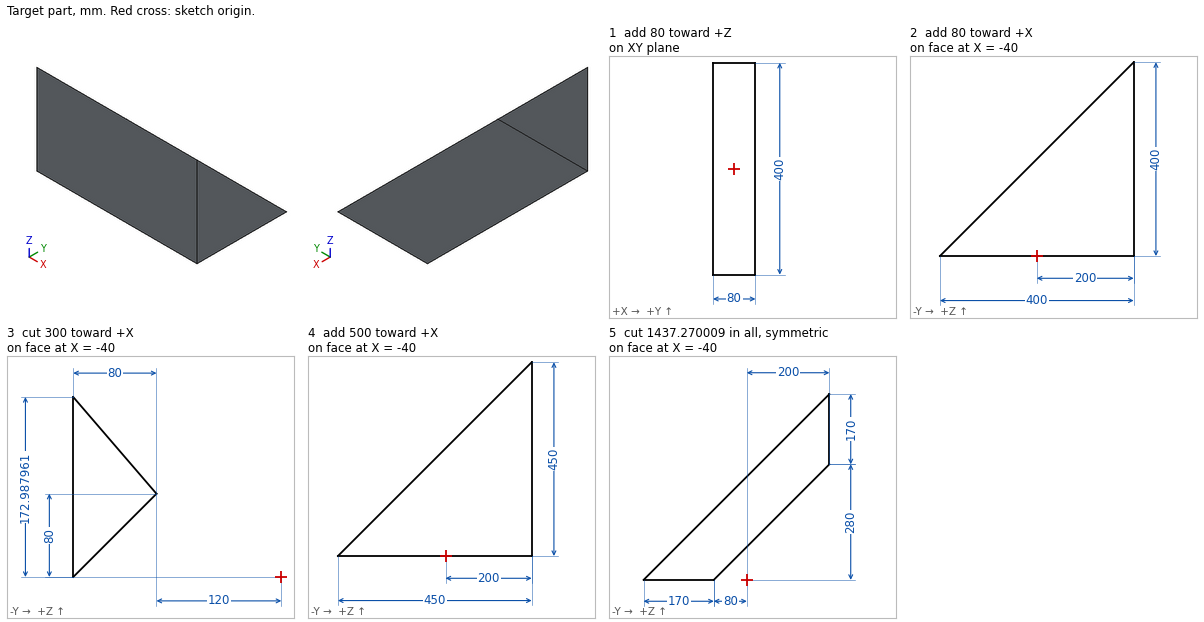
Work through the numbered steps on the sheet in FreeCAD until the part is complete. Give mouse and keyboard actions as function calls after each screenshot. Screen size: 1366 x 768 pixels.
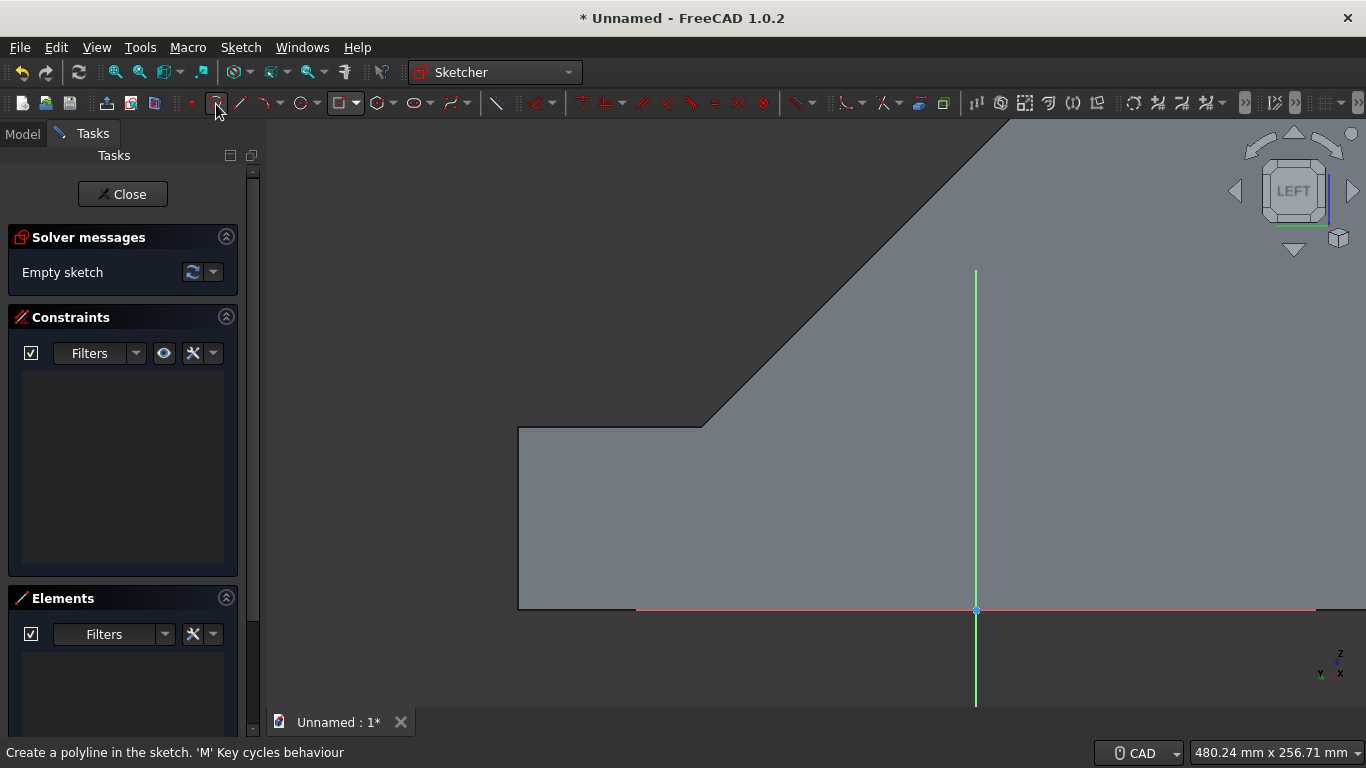
click(701, 427)
click(518, 214)
click(518, 610)
click(701, 428)
key(Escape)
key(Escape)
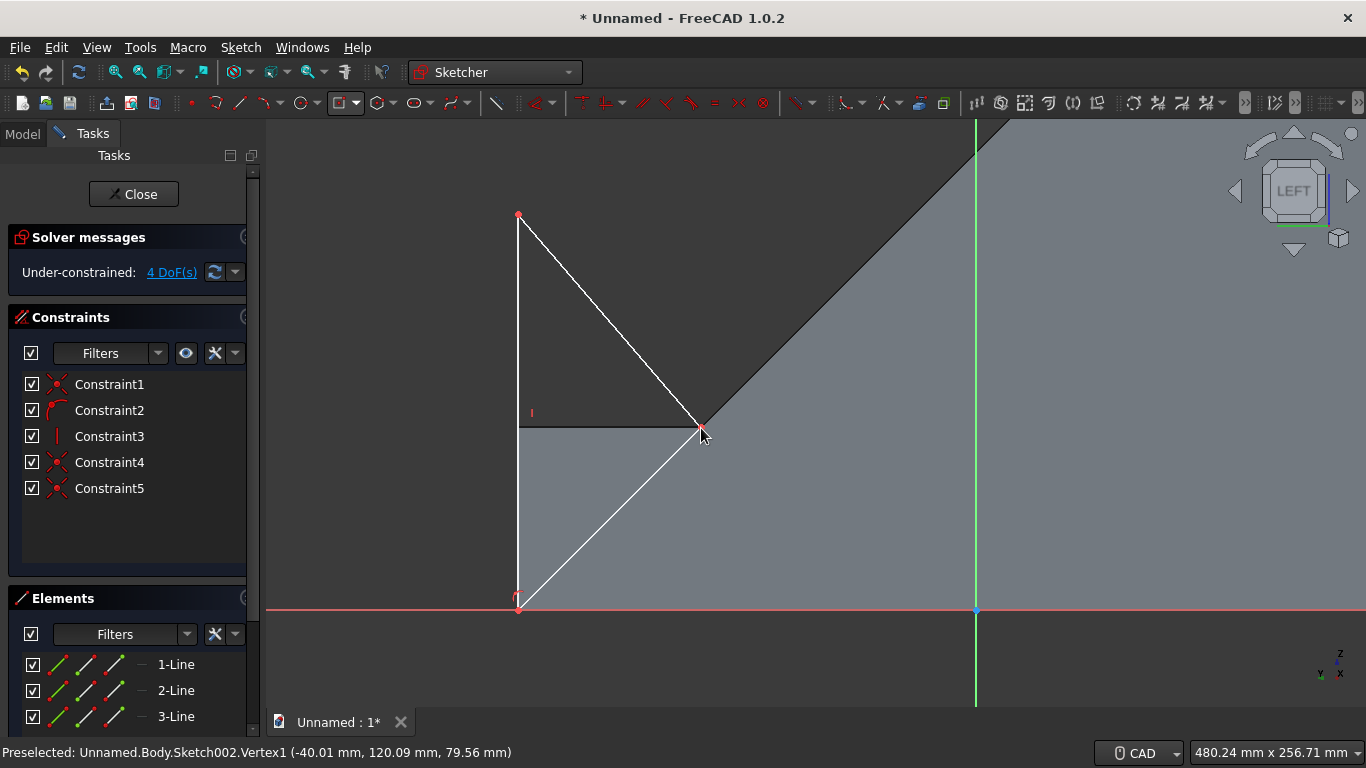
click(536, 104)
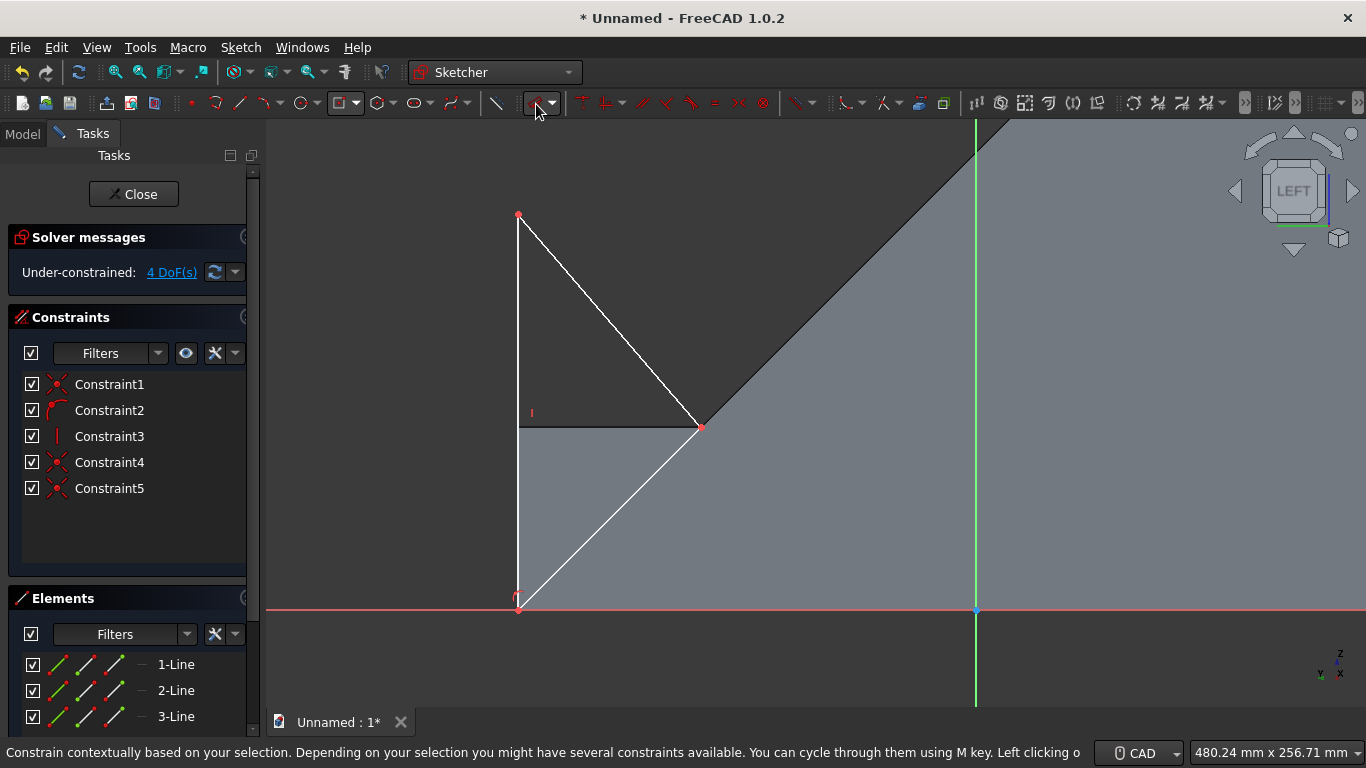
click(701, 428)
click(1010, 519)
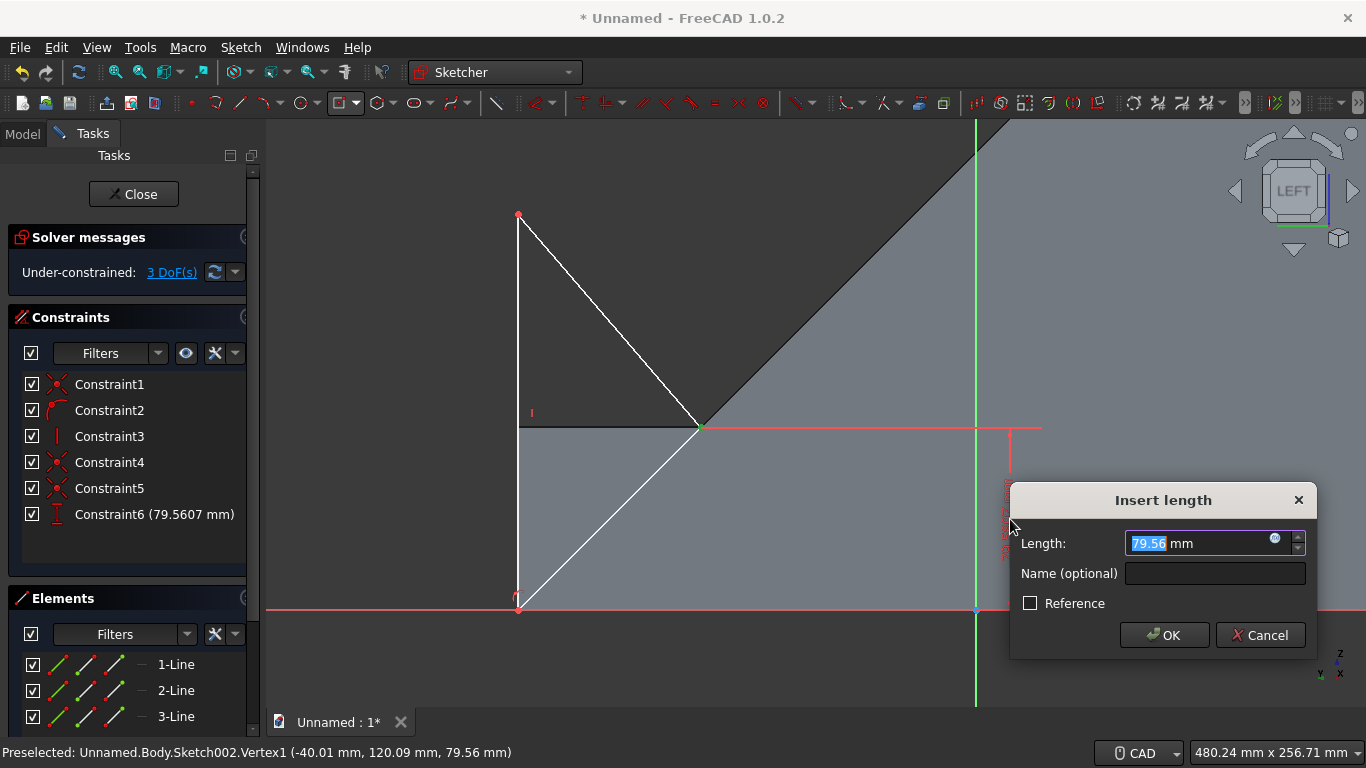
text(80)
key(Return)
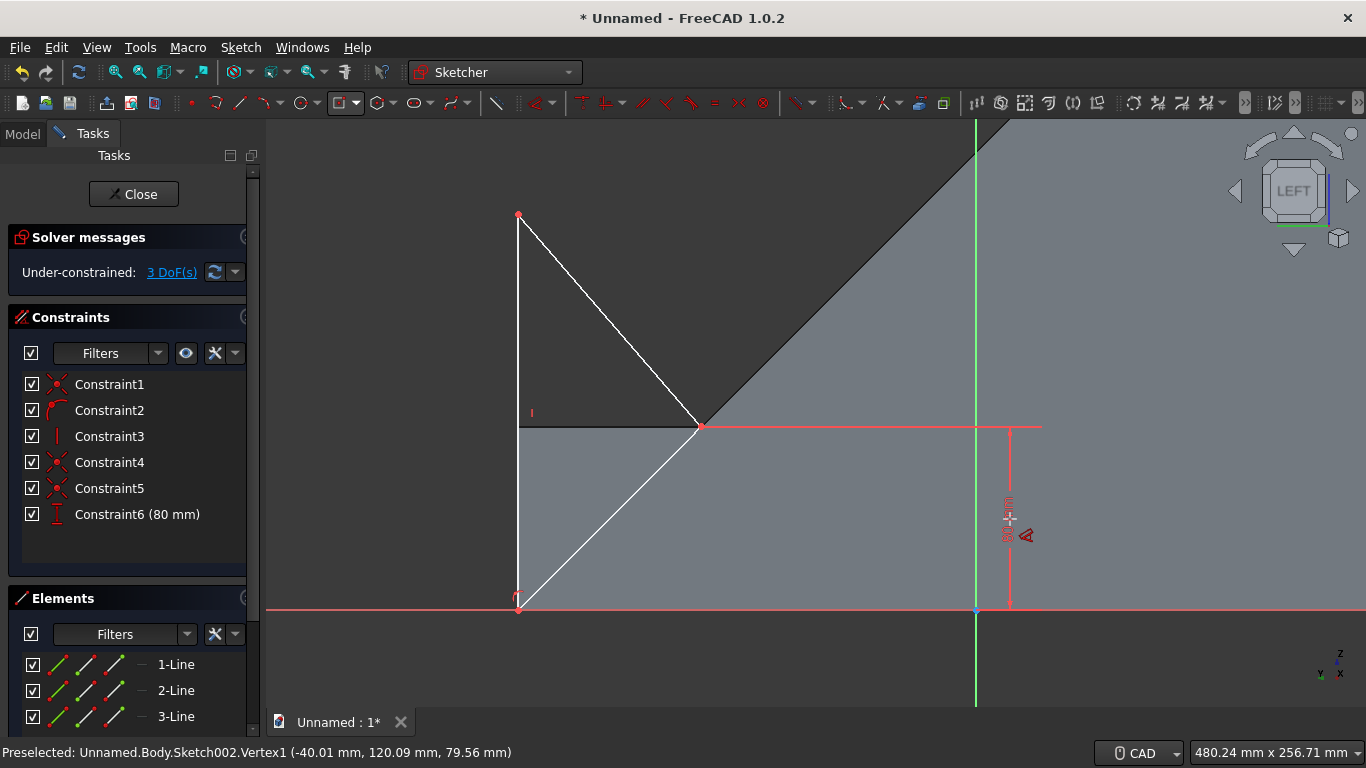
click(646, 363)
click(610, 181)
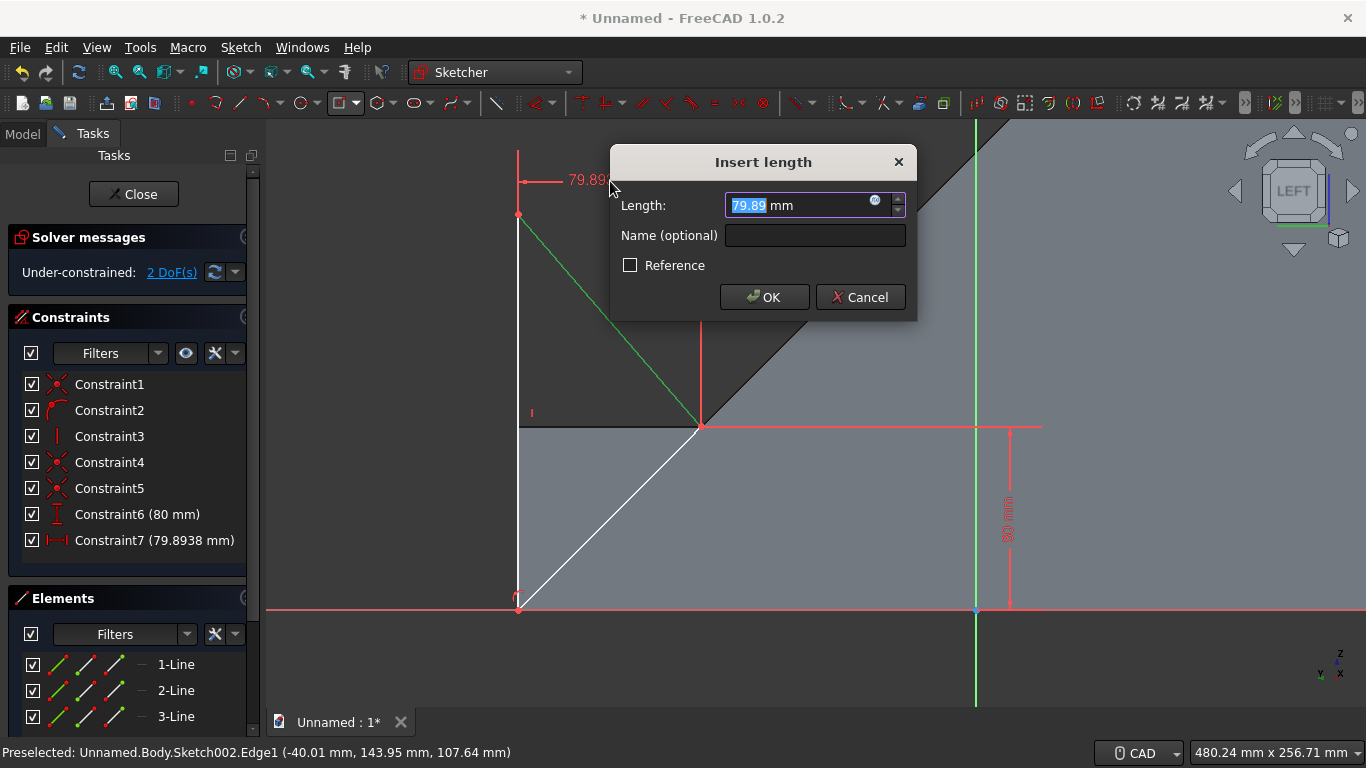
text(80)
key(Return)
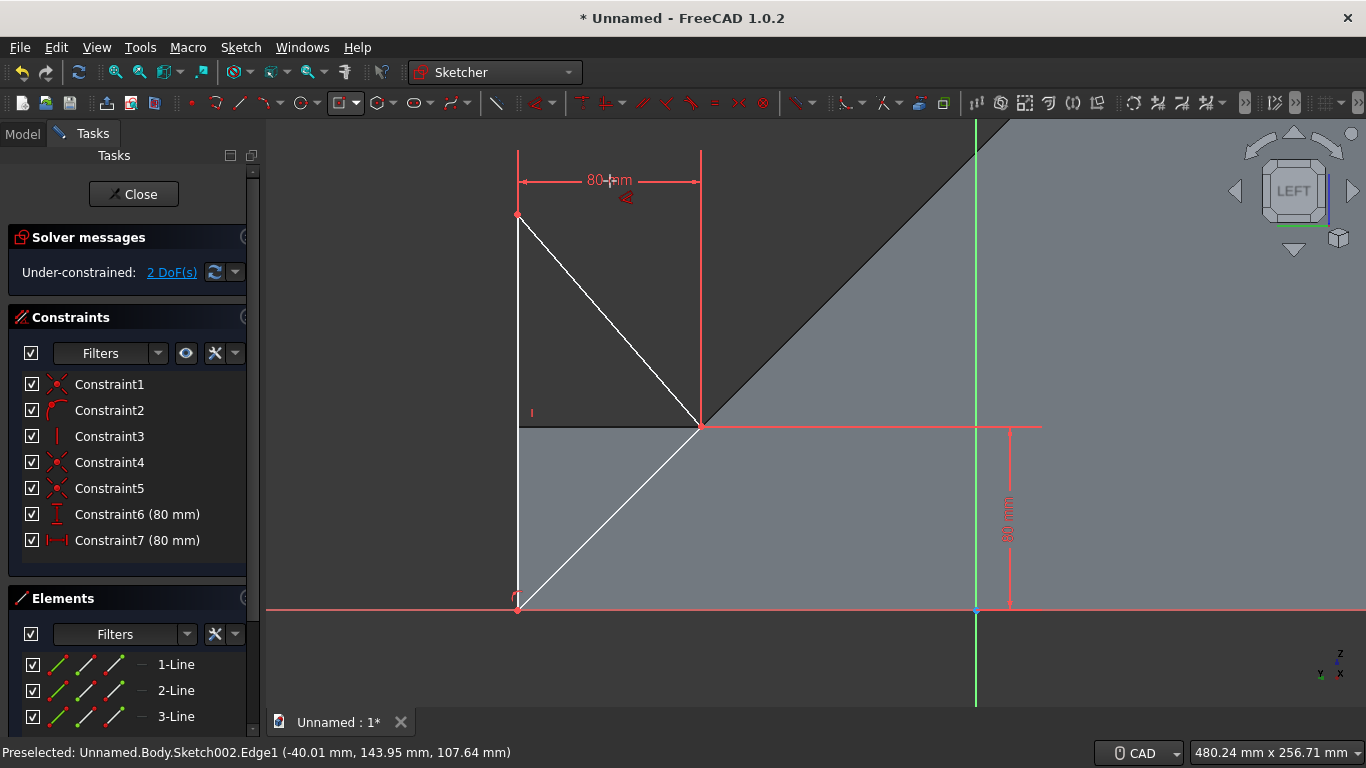
click(701, 427)
click(839, 644)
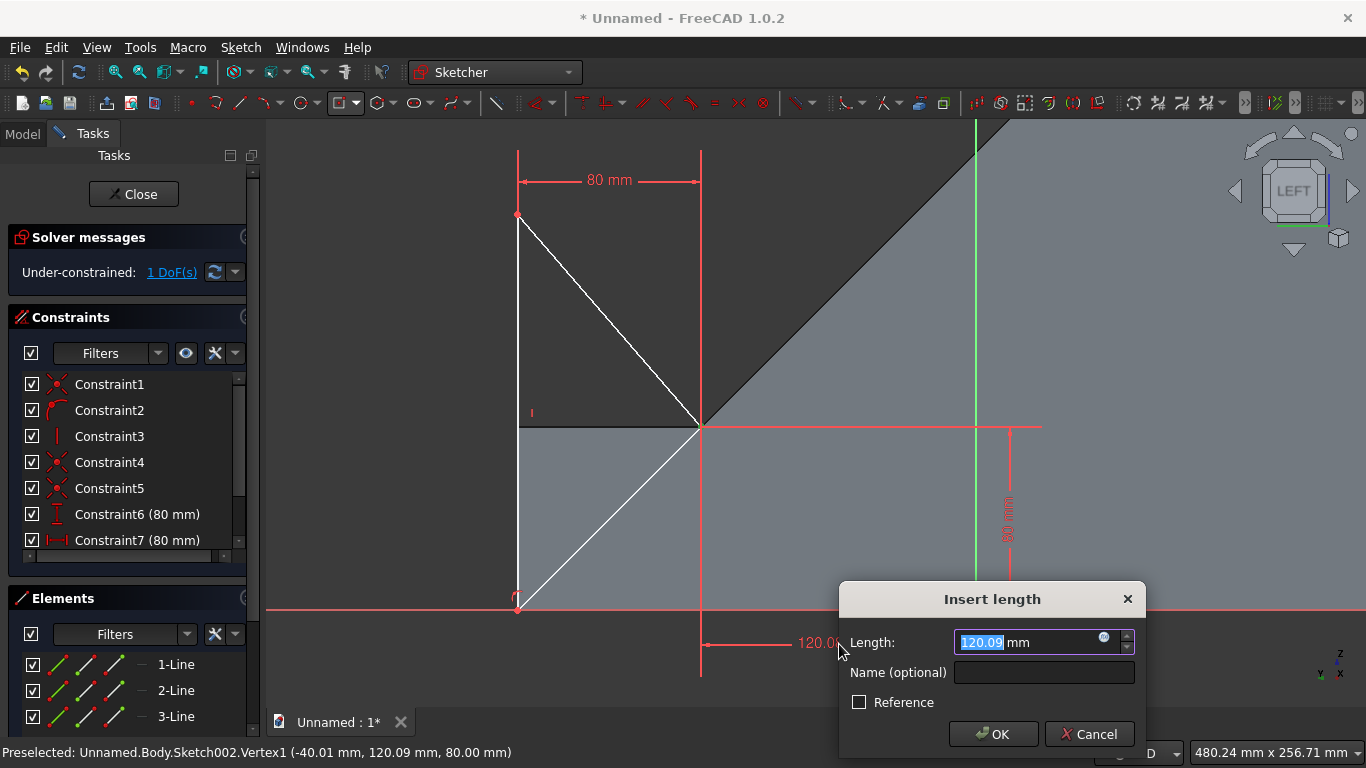
text(120)
key(Return)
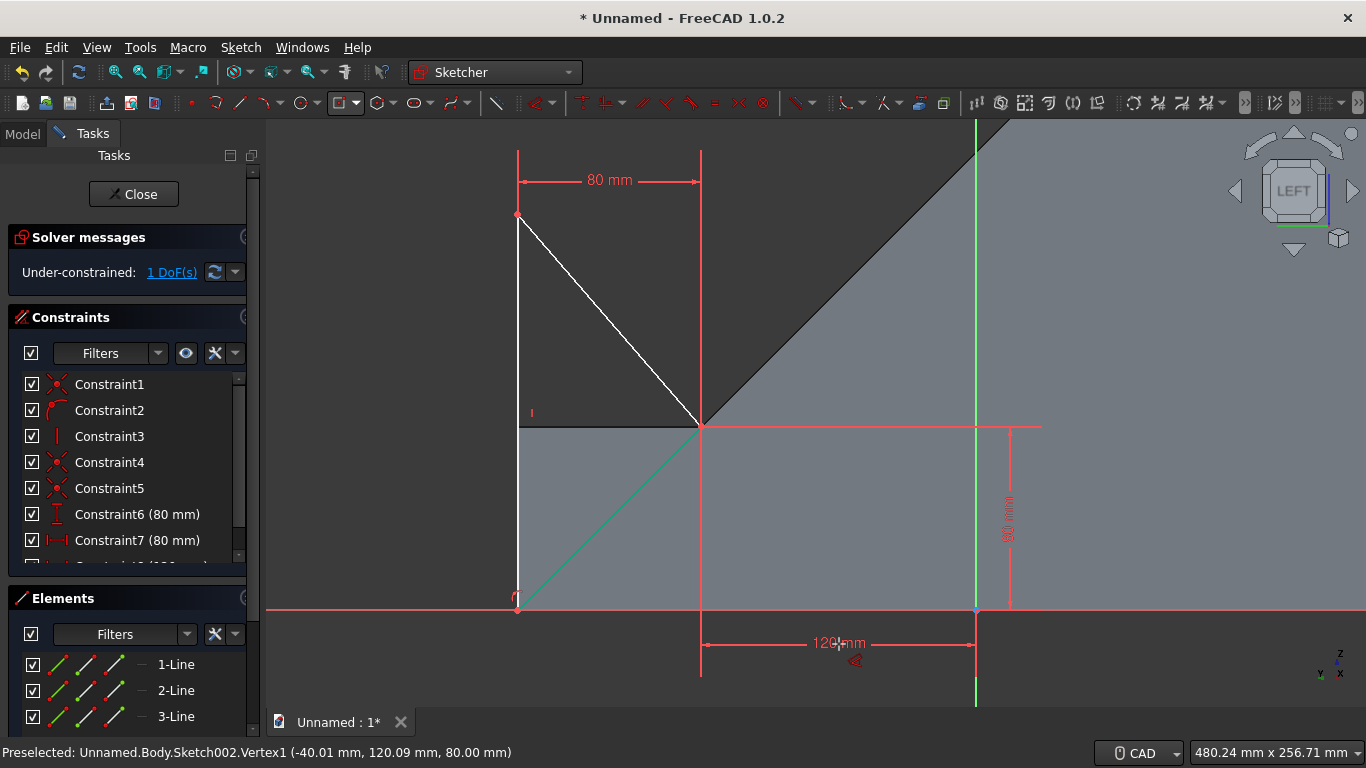
click(518, 334)
click(484, 413)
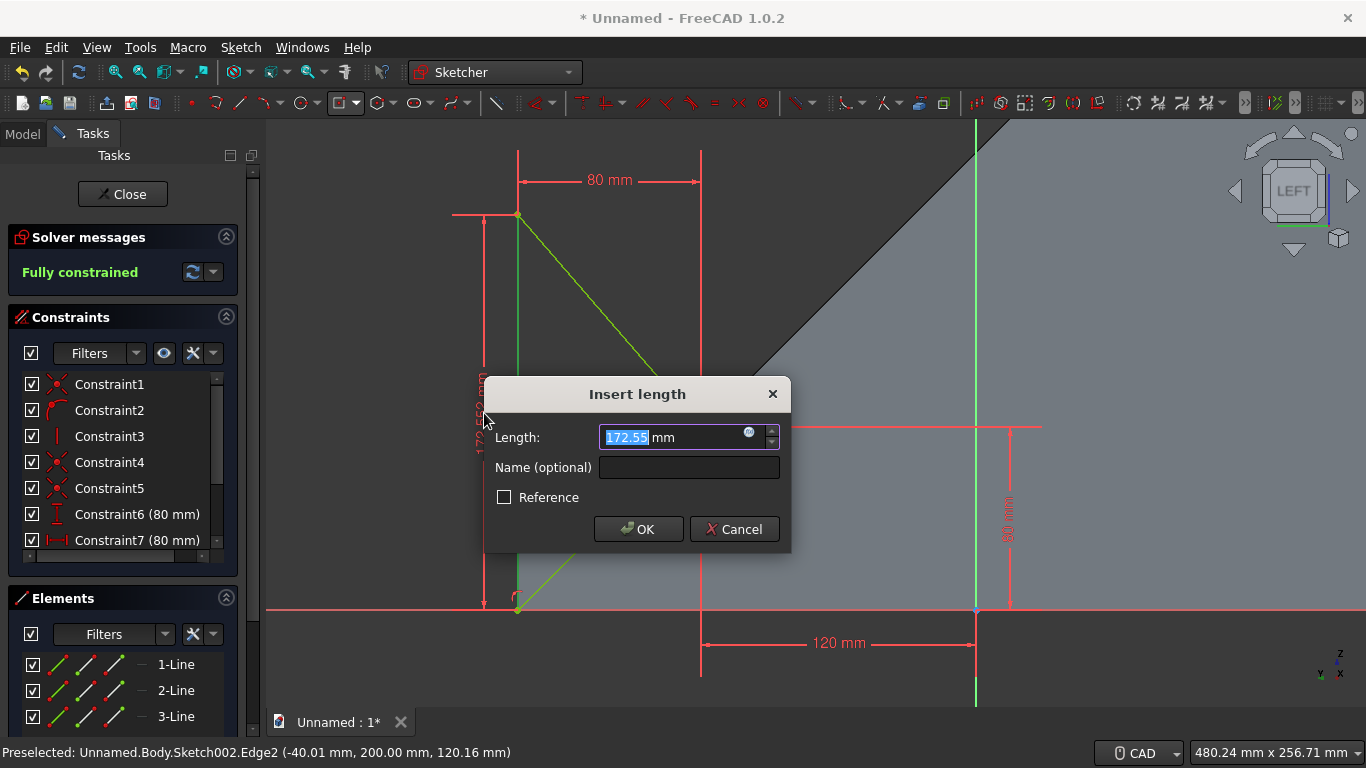
text(172.987961)
key(Return)
key(Escape)